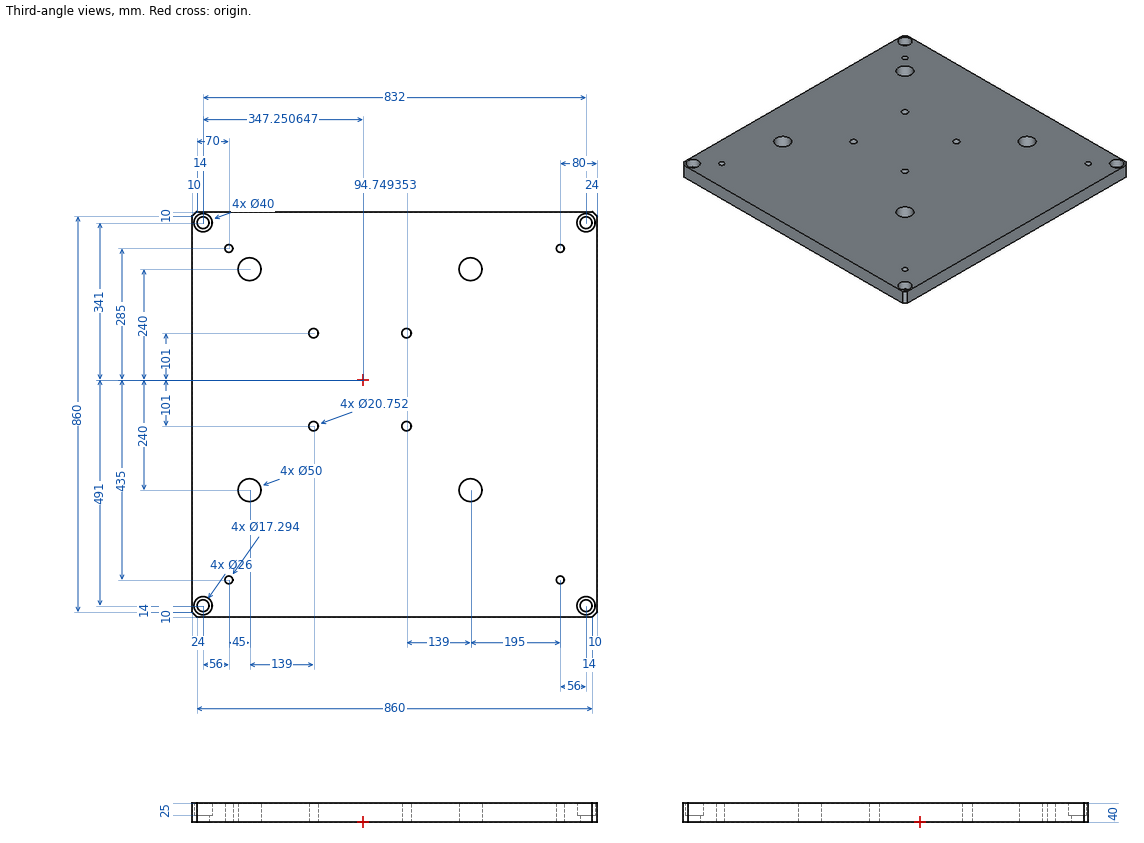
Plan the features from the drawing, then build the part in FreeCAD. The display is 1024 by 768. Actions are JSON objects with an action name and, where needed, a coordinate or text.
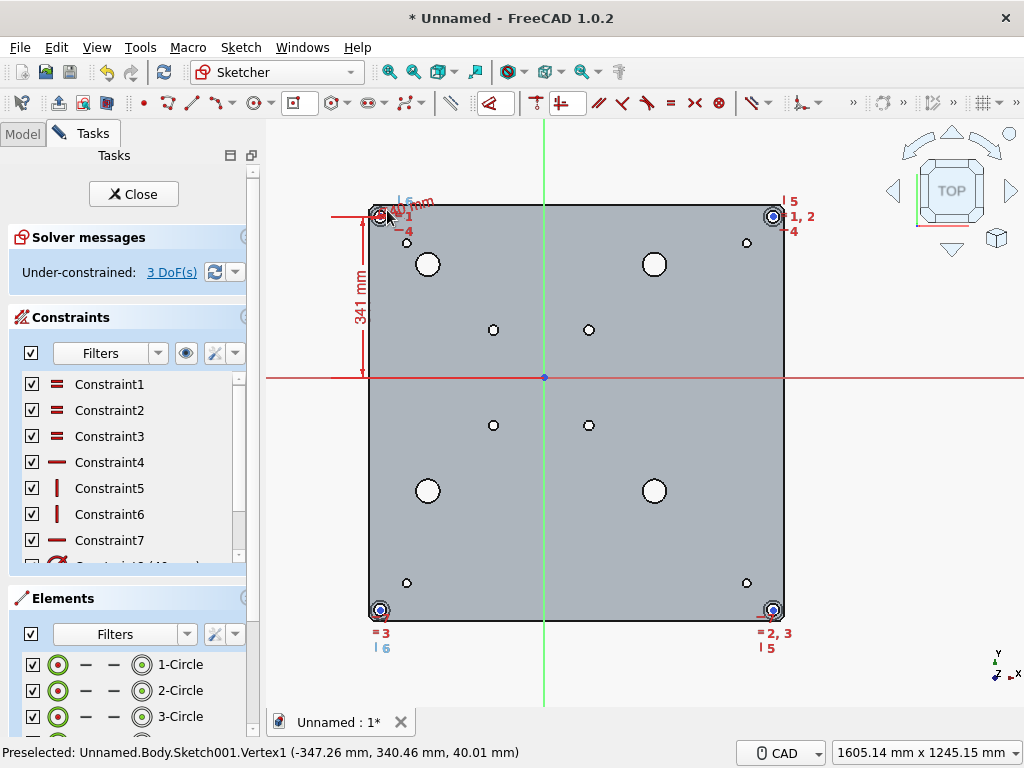
{"action": "left_click", "coordinate": [773, 610]}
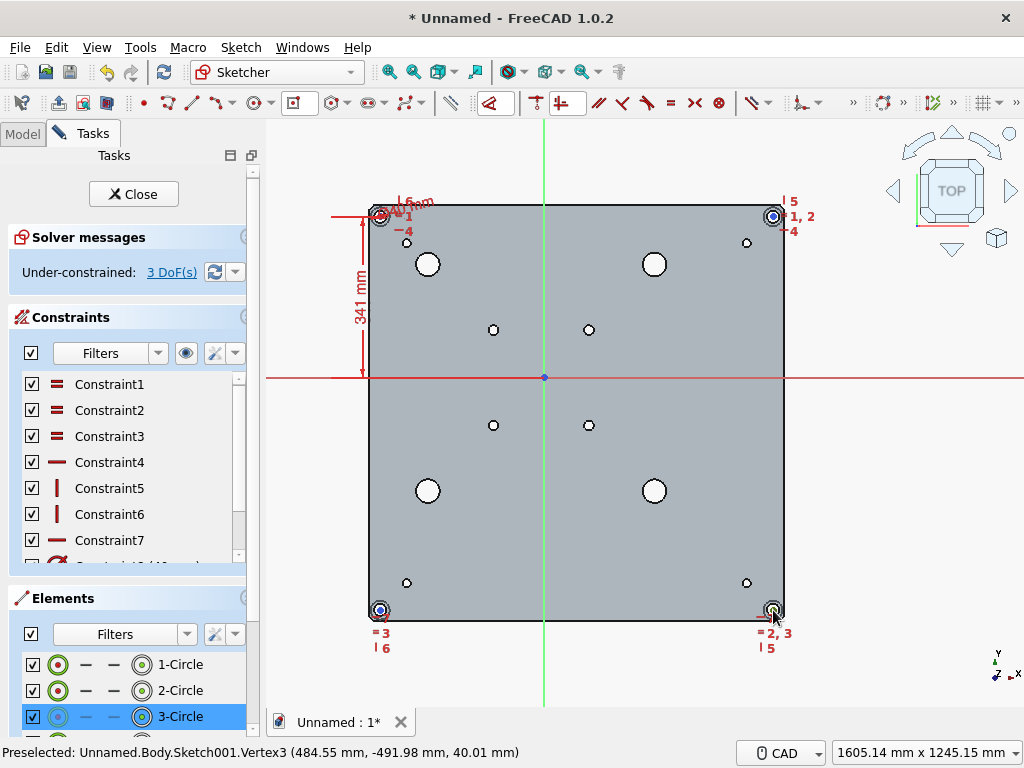
{"action": "left_click", "coordinate": [508, 104]}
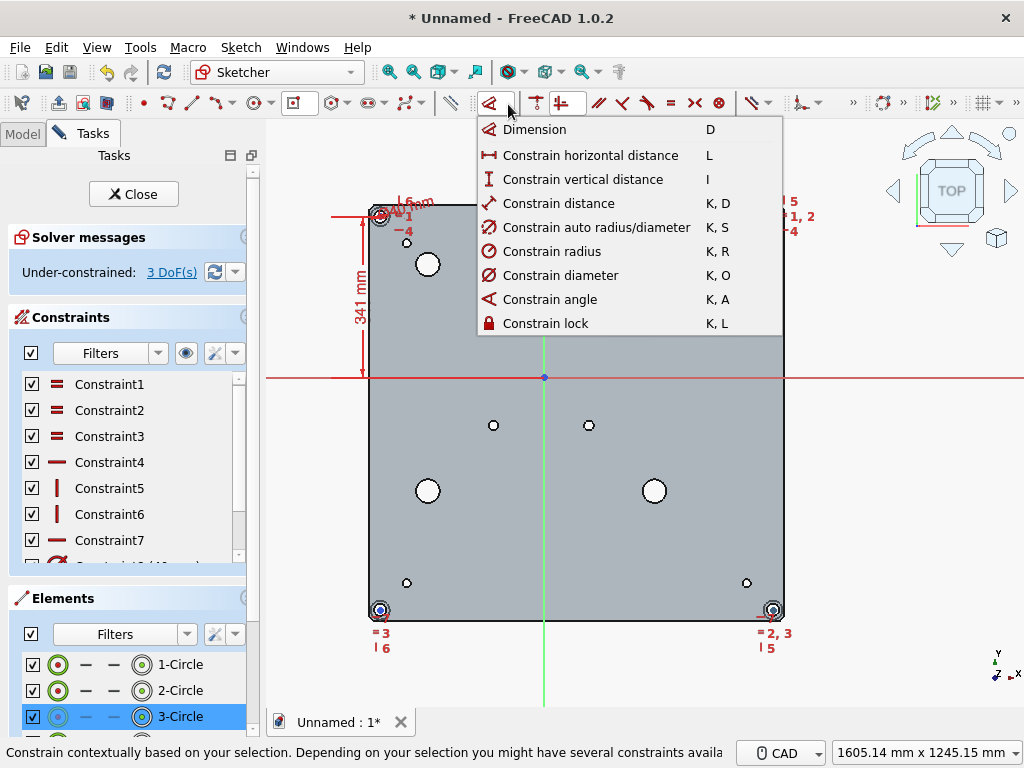
{"action": "left_click", "coordinate": [630, 179]}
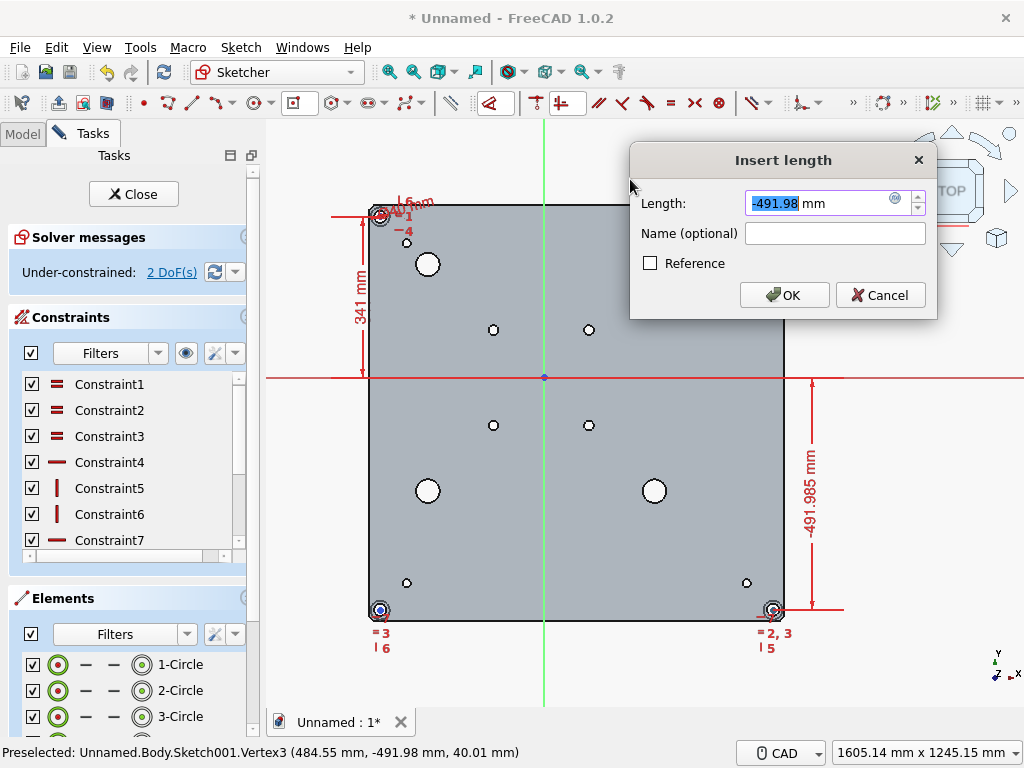
{"action": "type", "text": "-491"}
{"action": "key", "text": "Return"}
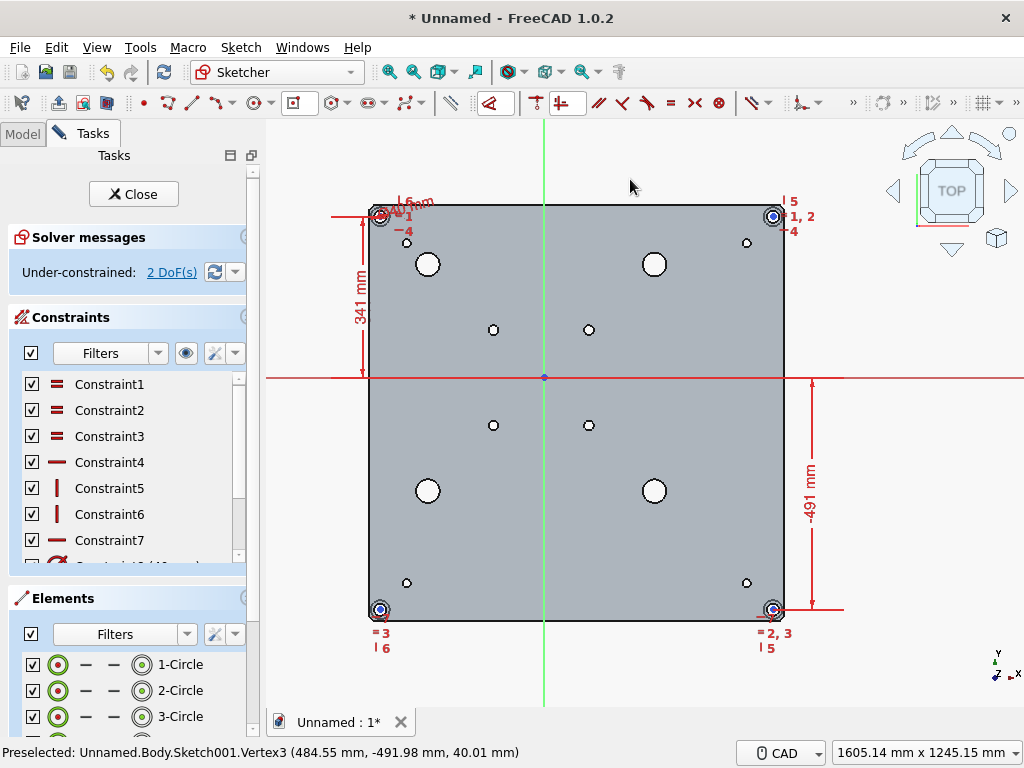
{"action": "left_click", "coordinate": [380, 217]}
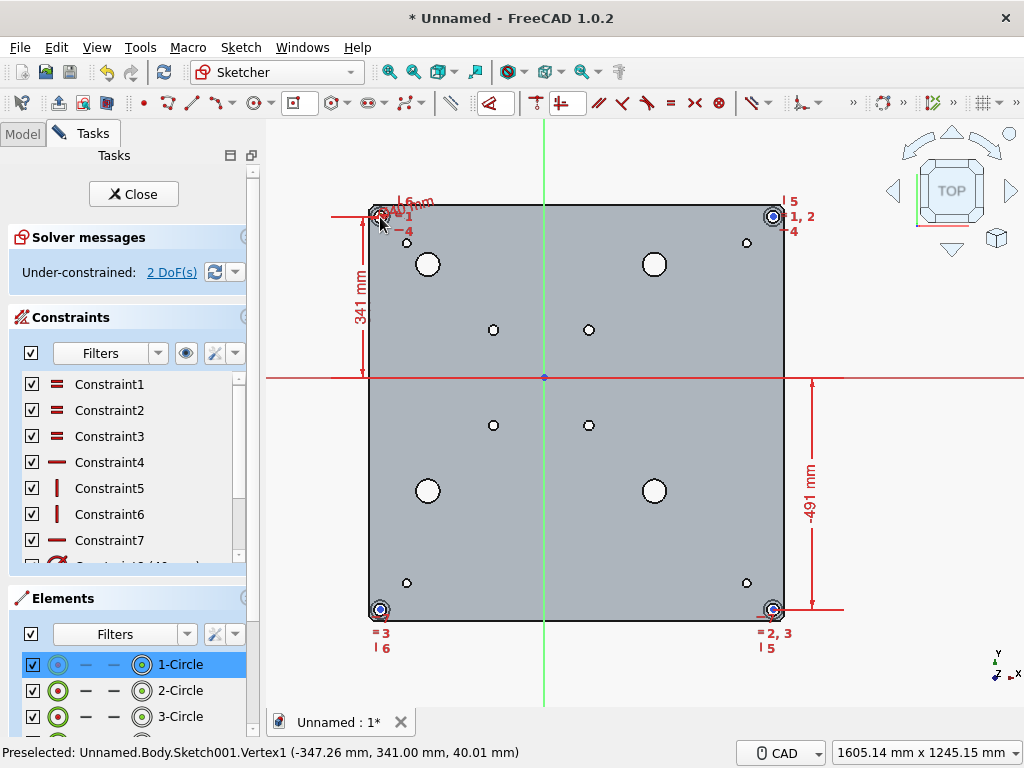
{"action": "left_click", "coordinate": [773, 217]}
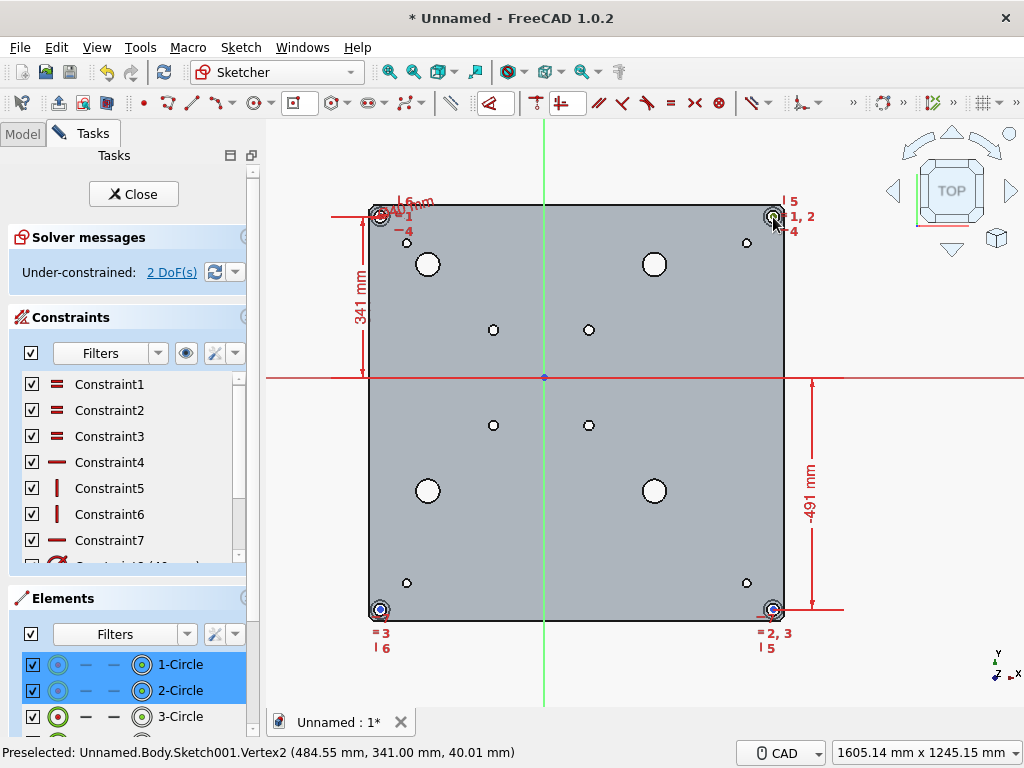
{"action": "key", "text": "l"}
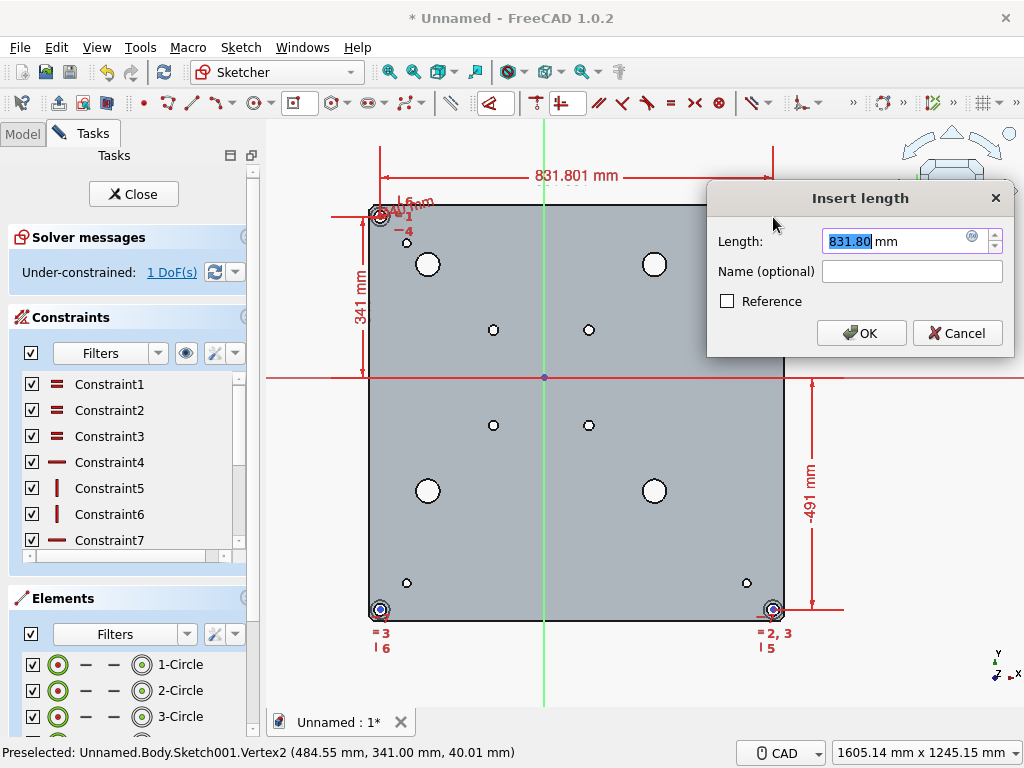
{"action": "type", "text": "832"}
{"action": "key", "text": "Return"}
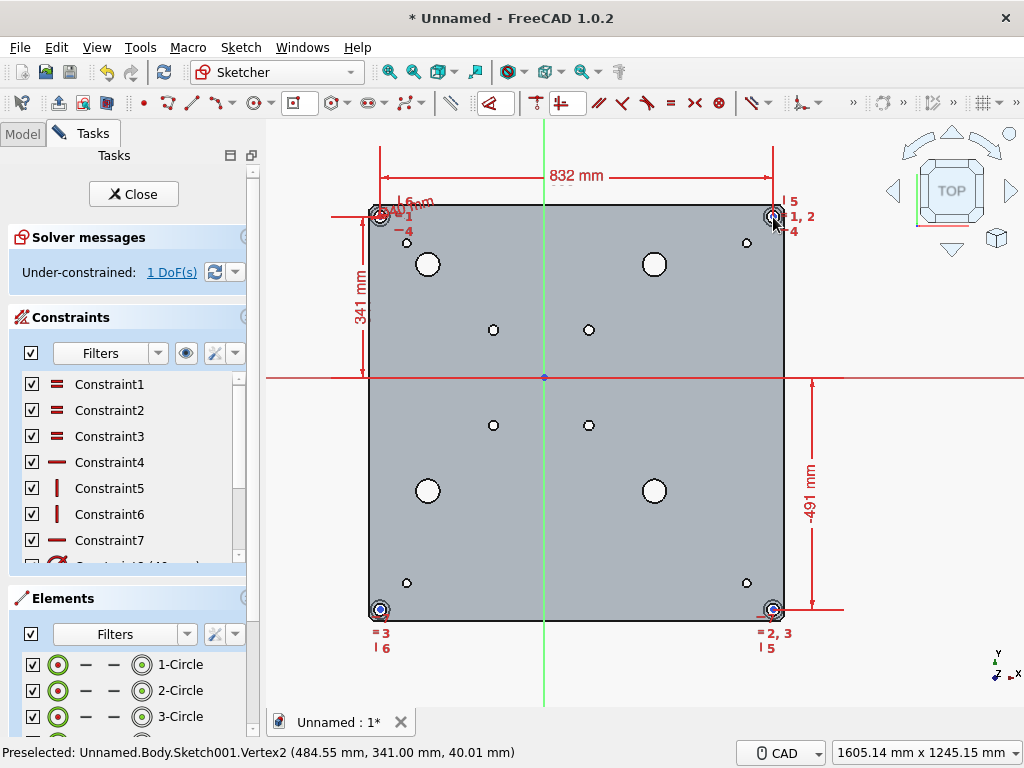
{"action": "left_click", "coordinate": [380, 217]}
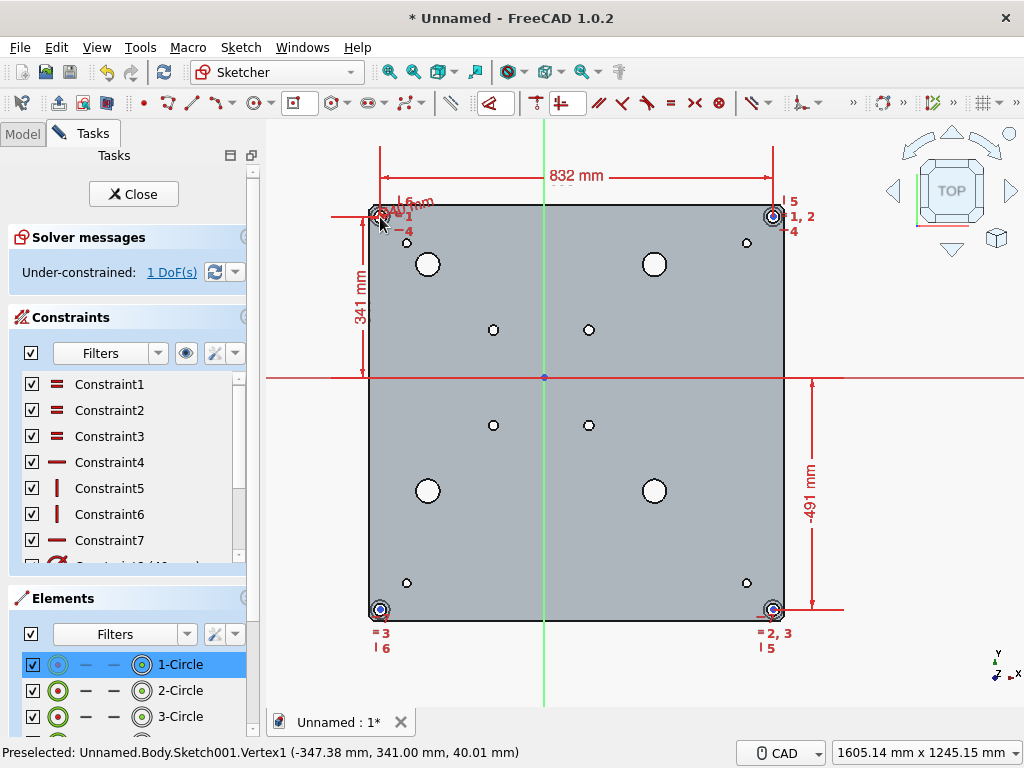
{"action": "key", "text": "l"}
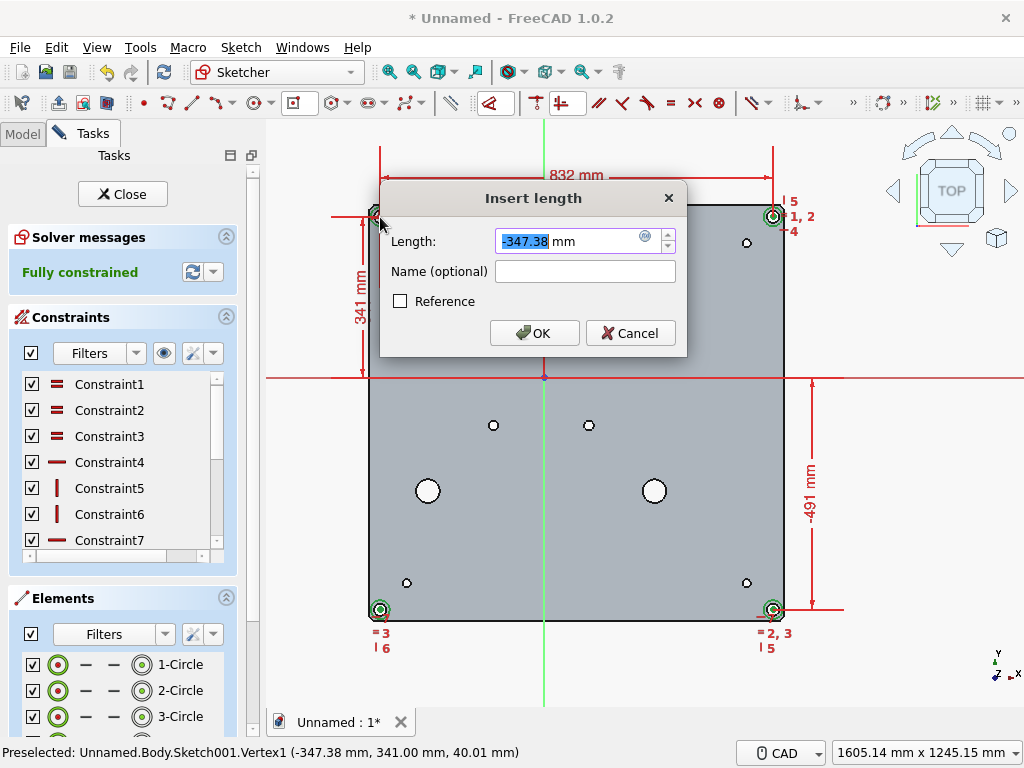
{"action": "type", "text": "-347.250647"}
{"action": "key", "text": "Return"}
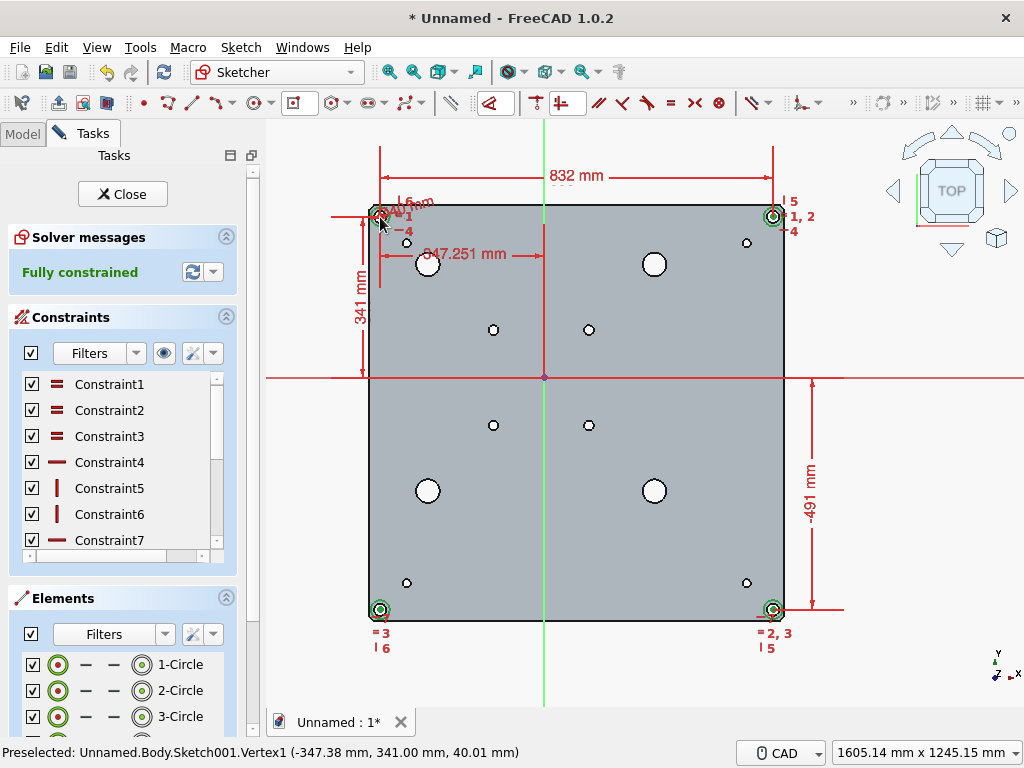
{"action": "left_click", "coordinate": [123, 194]}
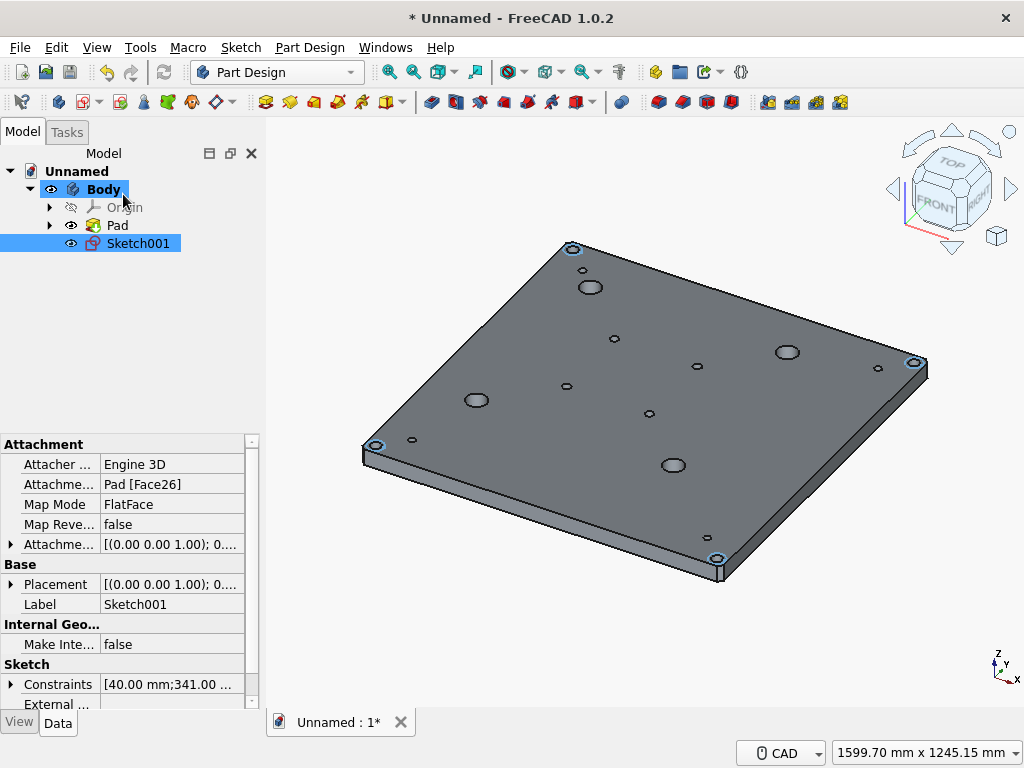
{"action": "left_click", "coordinate": [432, 102]}